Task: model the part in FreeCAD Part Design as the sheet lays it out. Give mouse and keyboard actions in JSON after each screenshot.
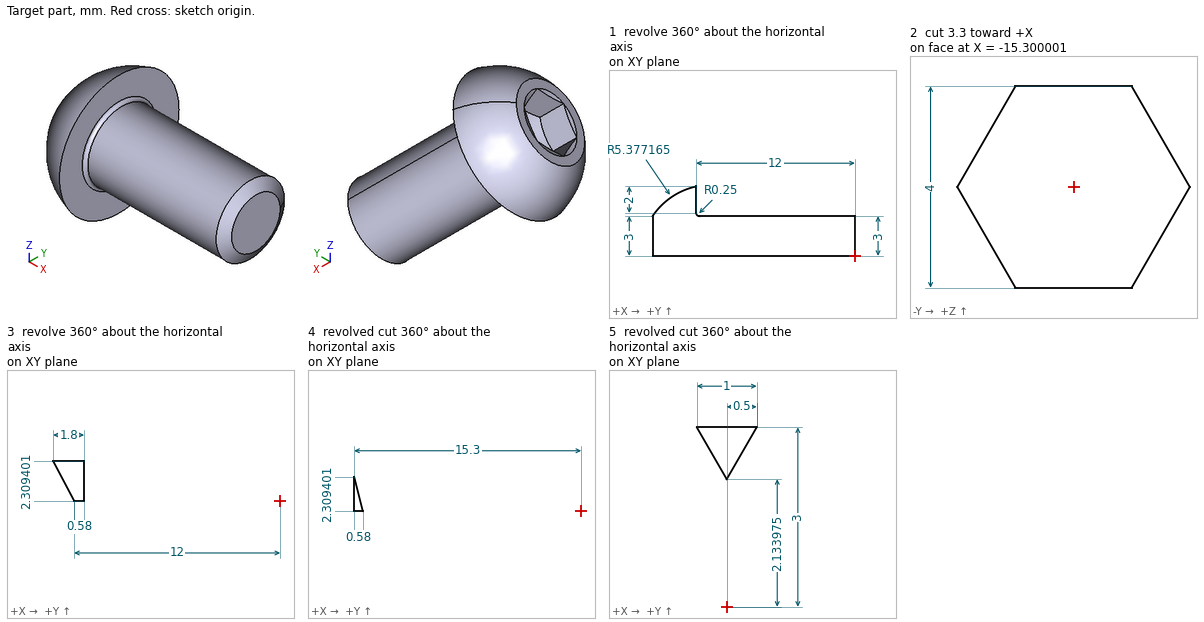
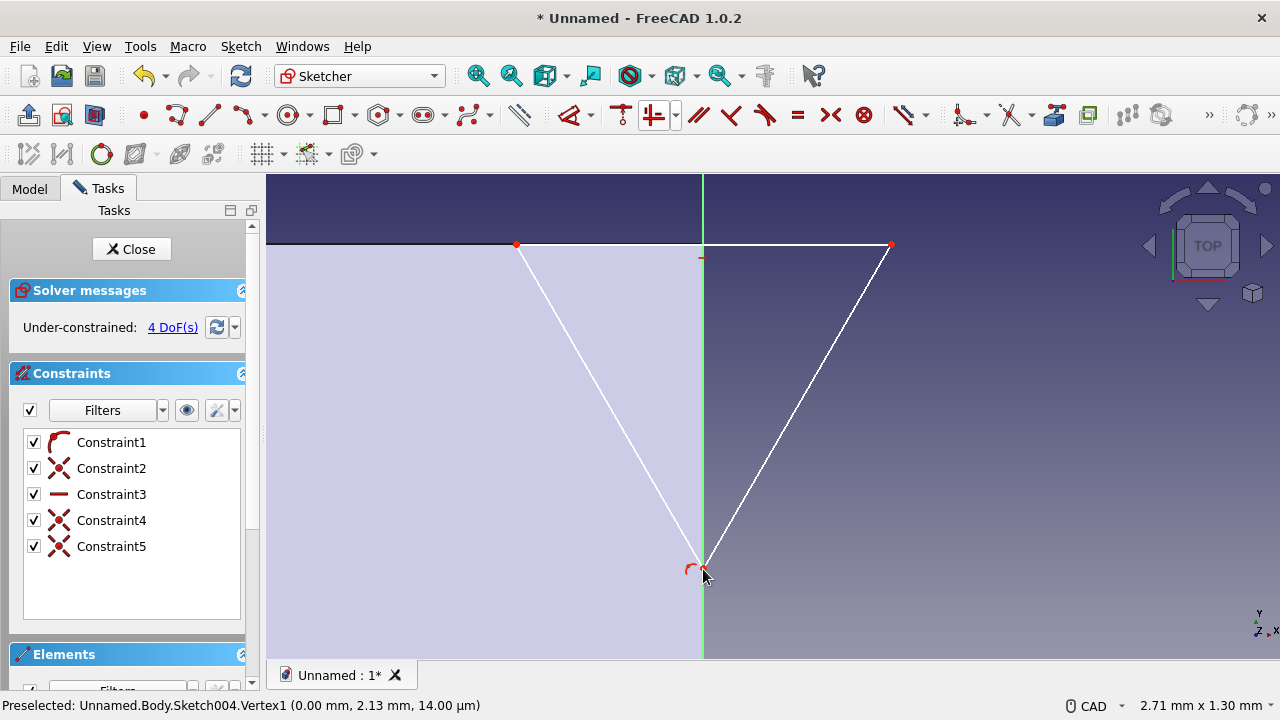
{"action": "left_click", "coordinate": [568, 116]}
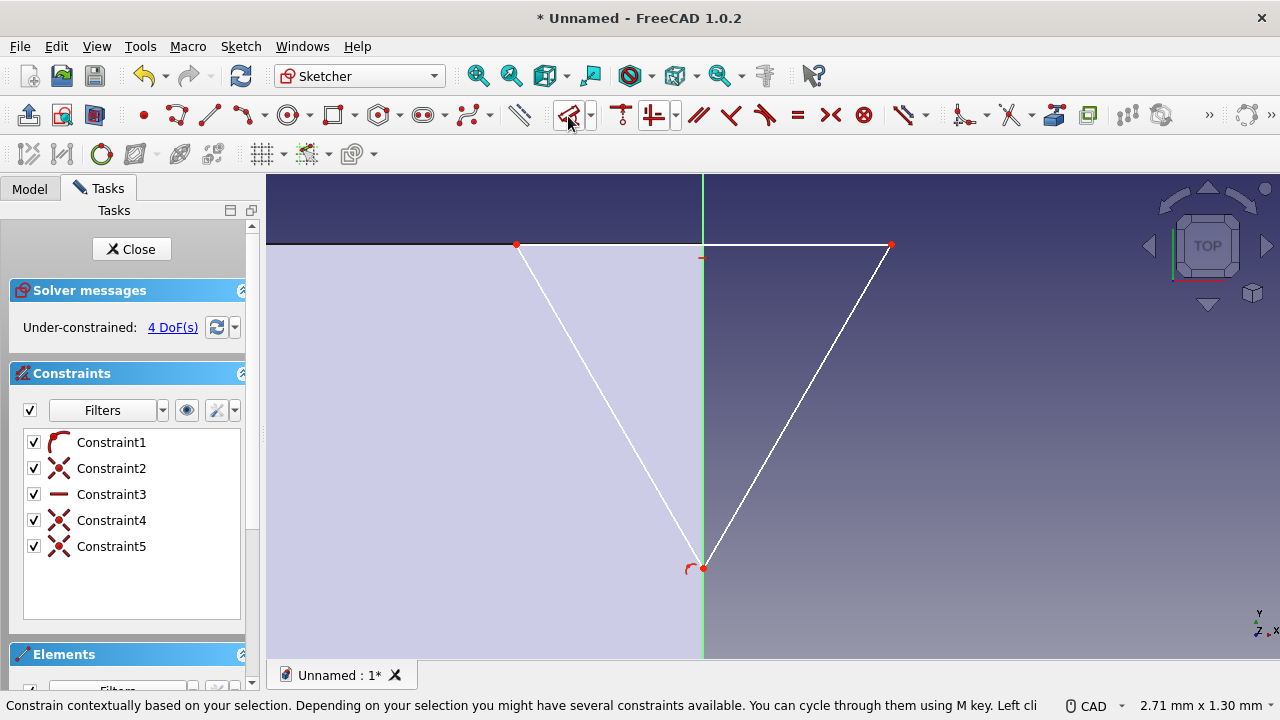
{"action": "left_click", "coordinate": [779, 245]}
{"action": "left_click", "coordinate": [617, 211]}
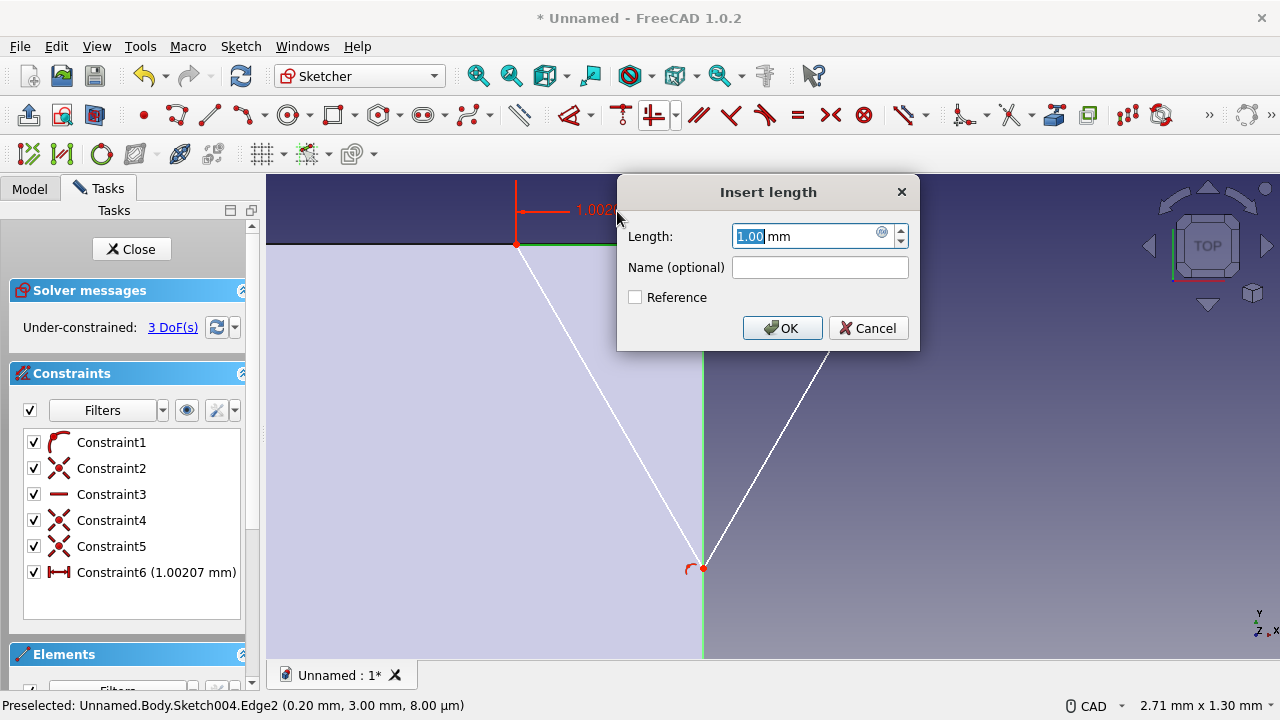
{"action": "type", "text": "1"}
{"action": "key", "text": "Return"}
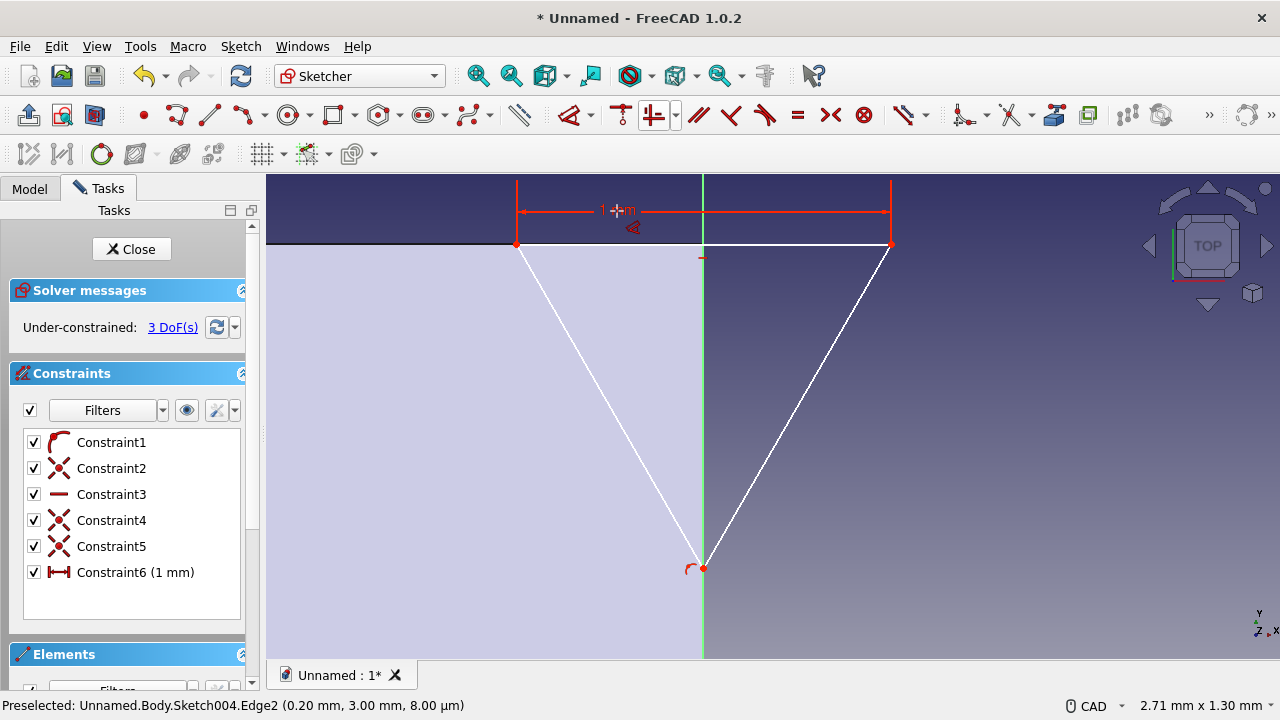
{"action": "left_click", "coordinate": [891, 245]}
{"action": "left_click", "coordinate": [925, 438]}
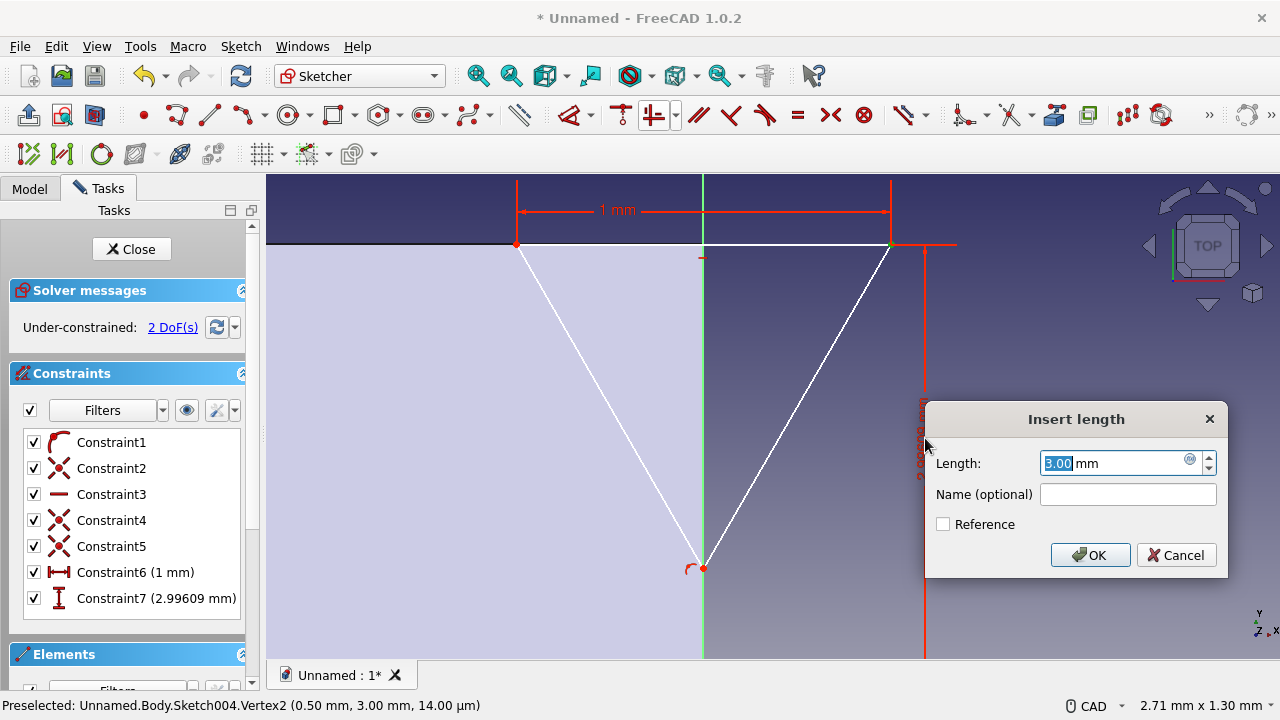
{"action": "type", "text": "3"}
{"action": "key", "text": "Return"}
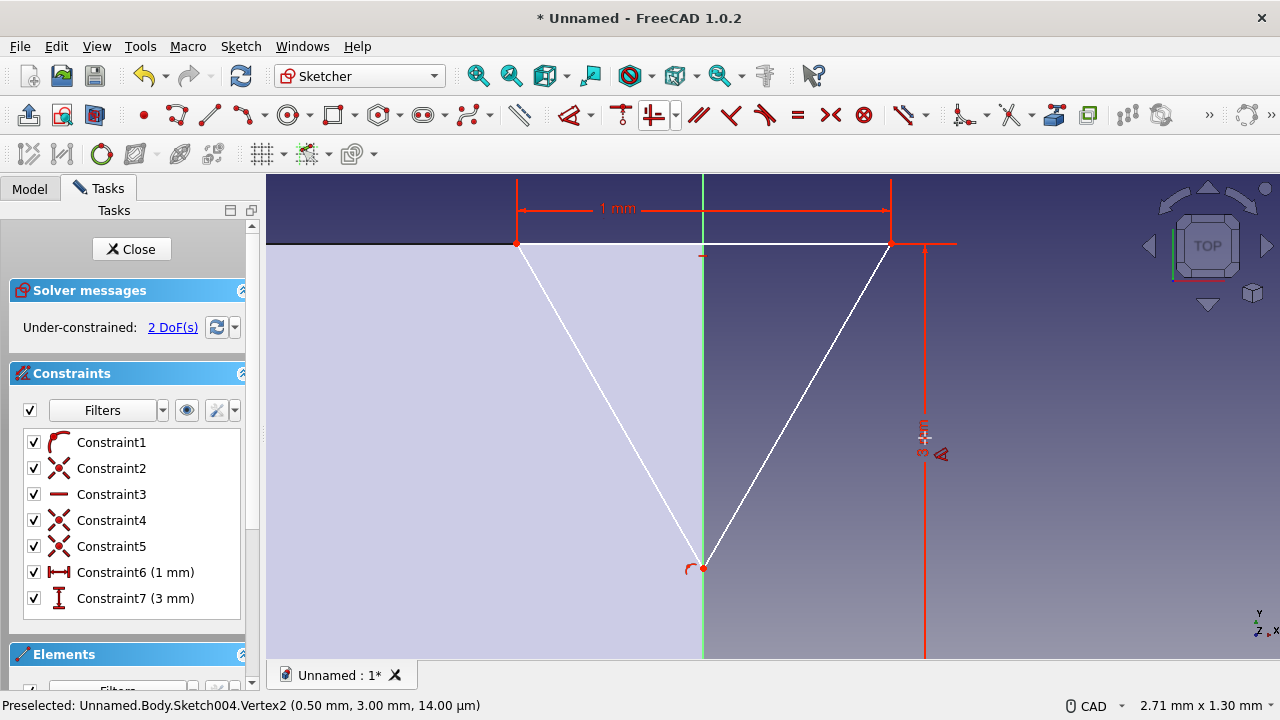
{"action": "left_click", "coordinate": [891, 244]}
{"action": "left_click", "coordinate": [797, 210]}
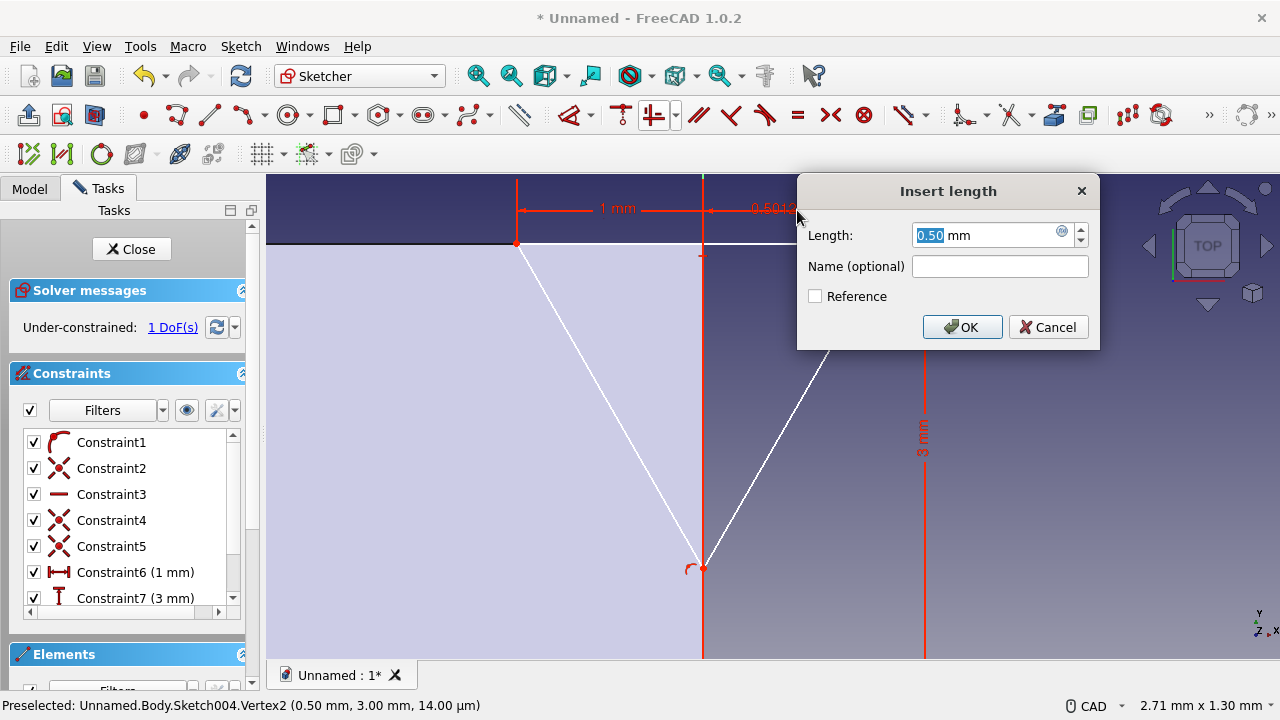
{"action": "type", "text": "0.5"}
{"action": "key", "text": "Return"}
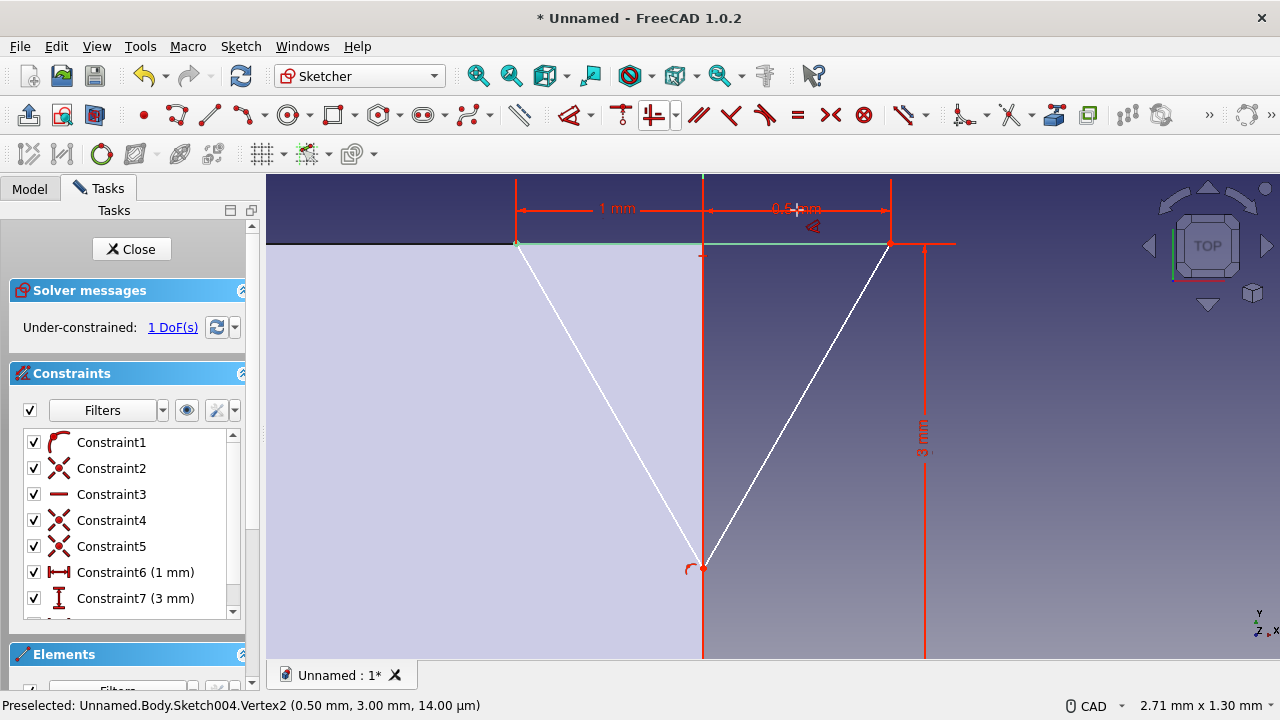
{"action": "left_click", "coordinate": [703, 569]}
{"action": "left_click", "coordinate": [737, 600]}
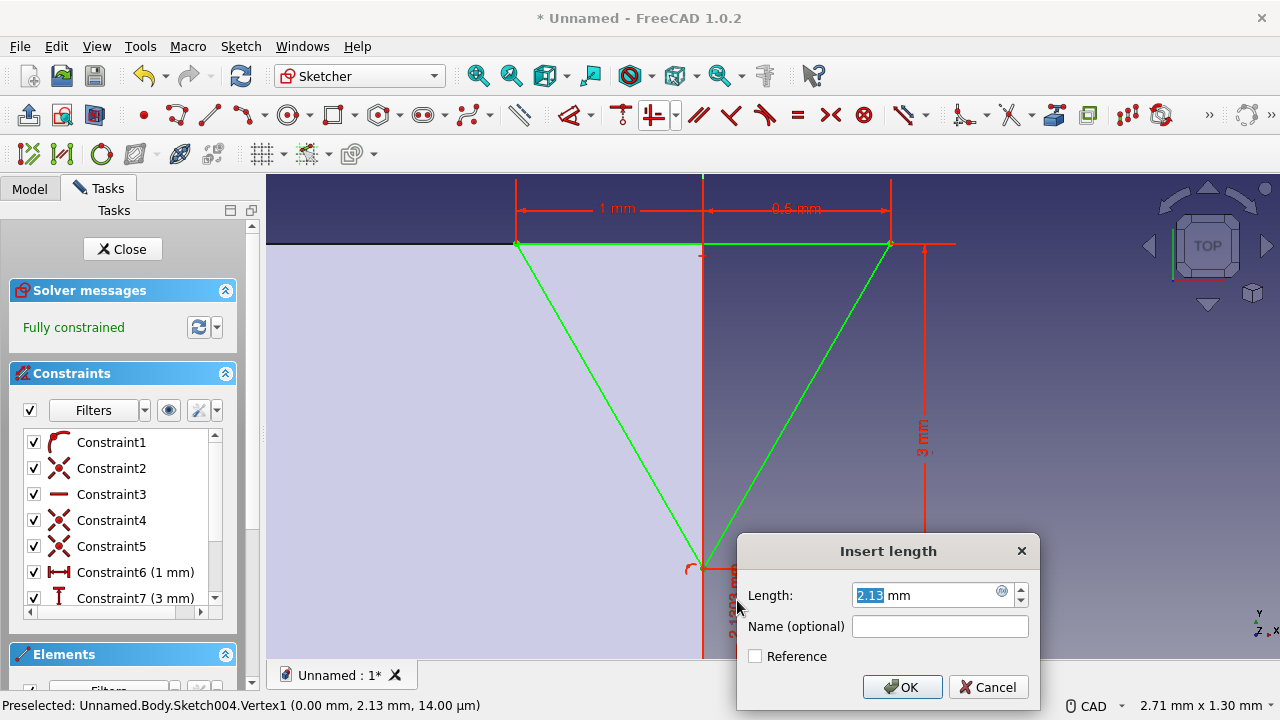
{"action": "type", "text": "2.133975"}
{"action": "key", "text": "Return"}
{"action": "key", "text": "Escape"}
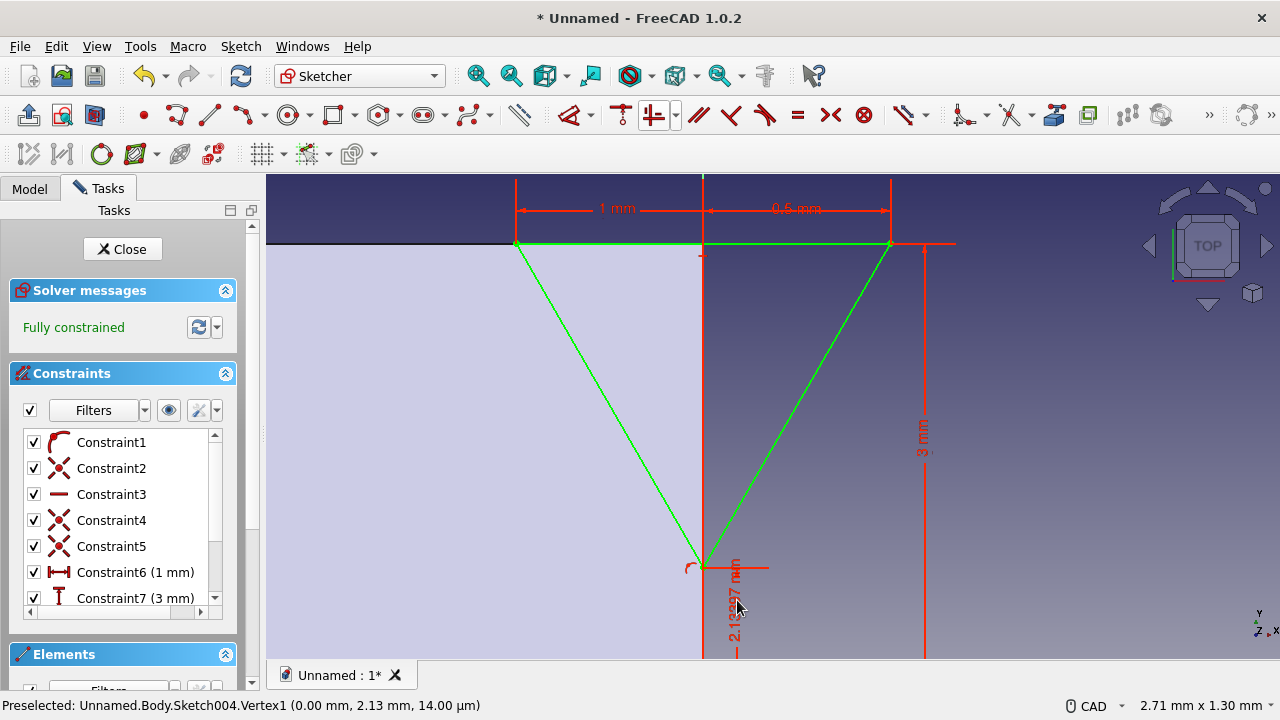
{"action": "left_click", "coordinate": [123, 249]}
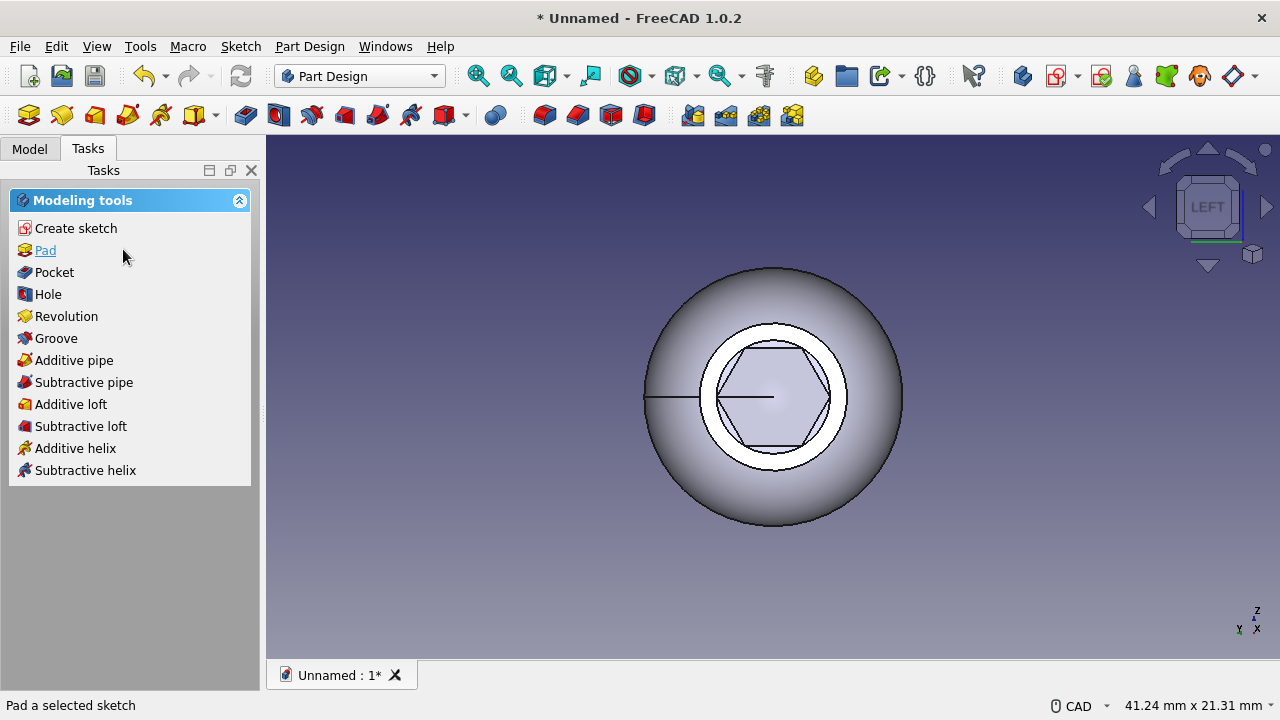
{"action": "left_click", "coordinate": [312, 116]}